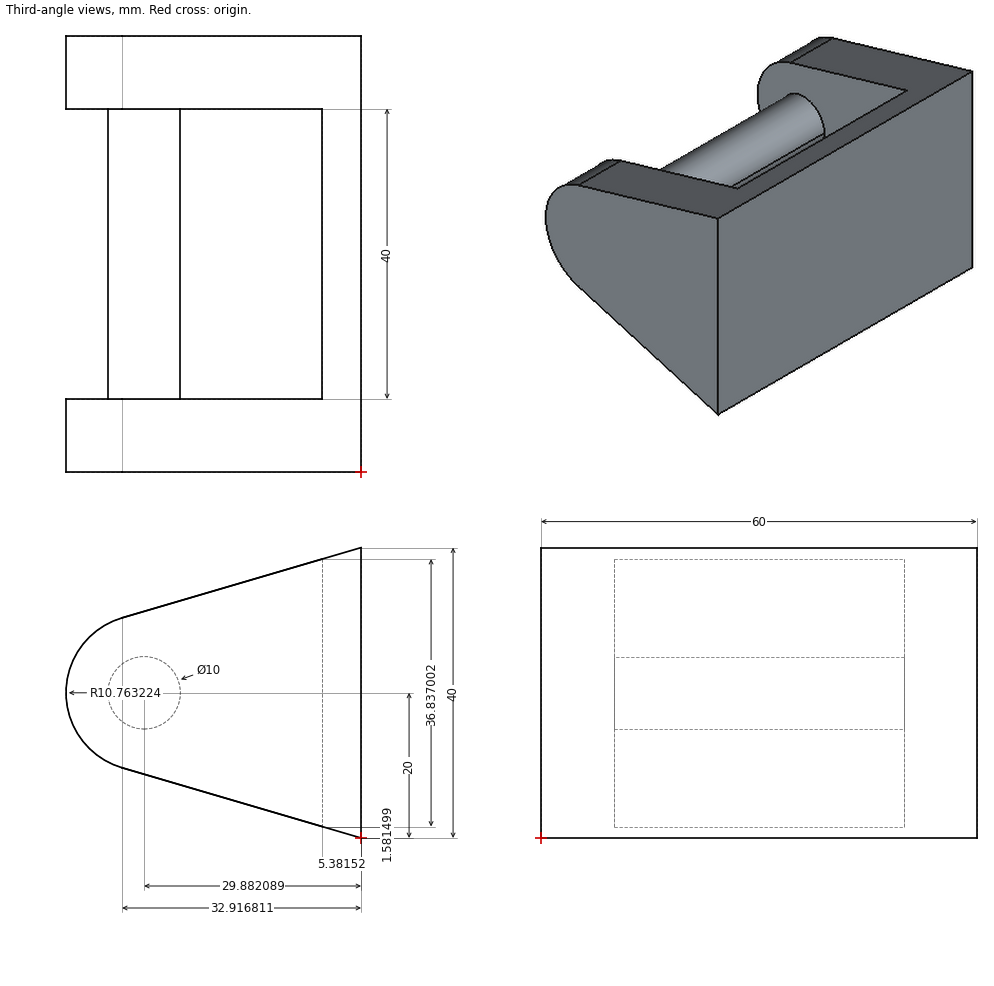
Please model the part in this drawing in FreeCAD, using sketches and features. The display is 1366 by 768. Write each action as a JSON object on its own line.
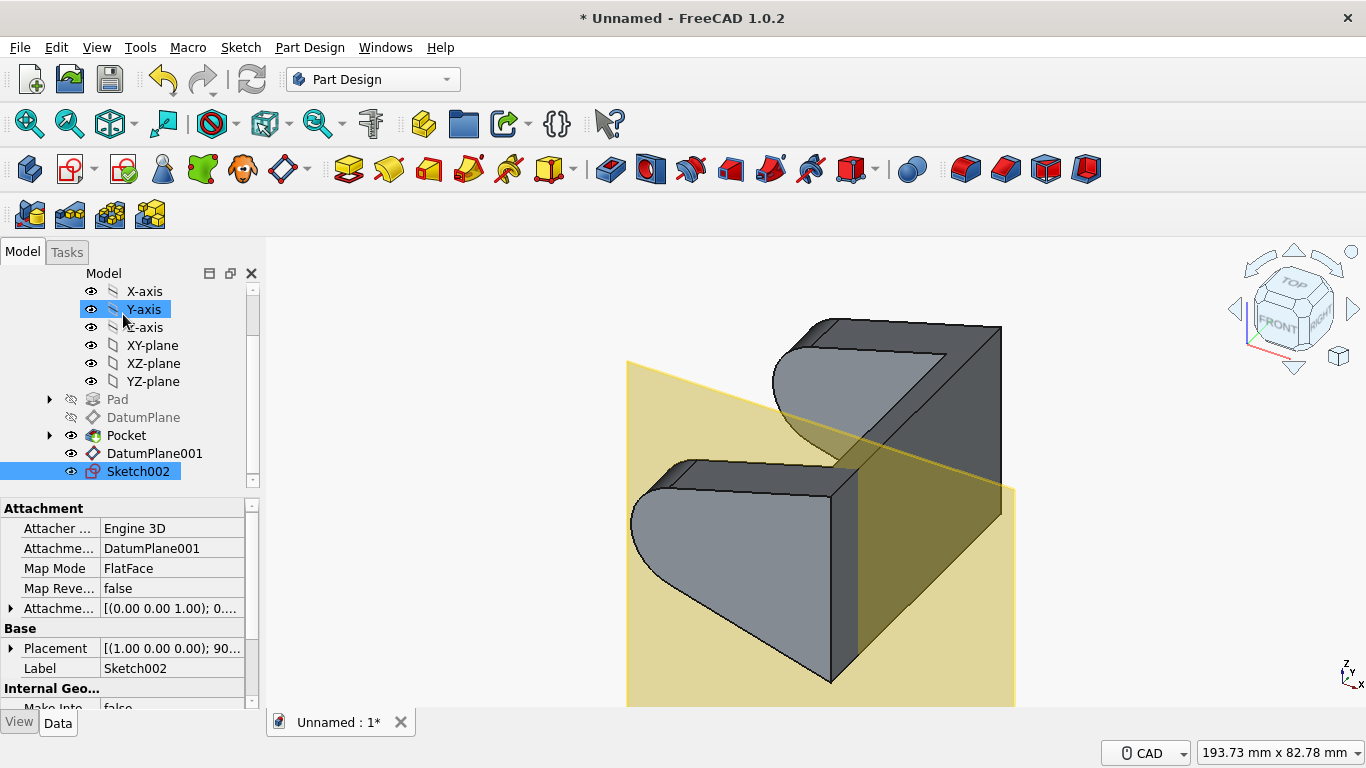
{"action": "left_click", "coordinate": [350, 170]}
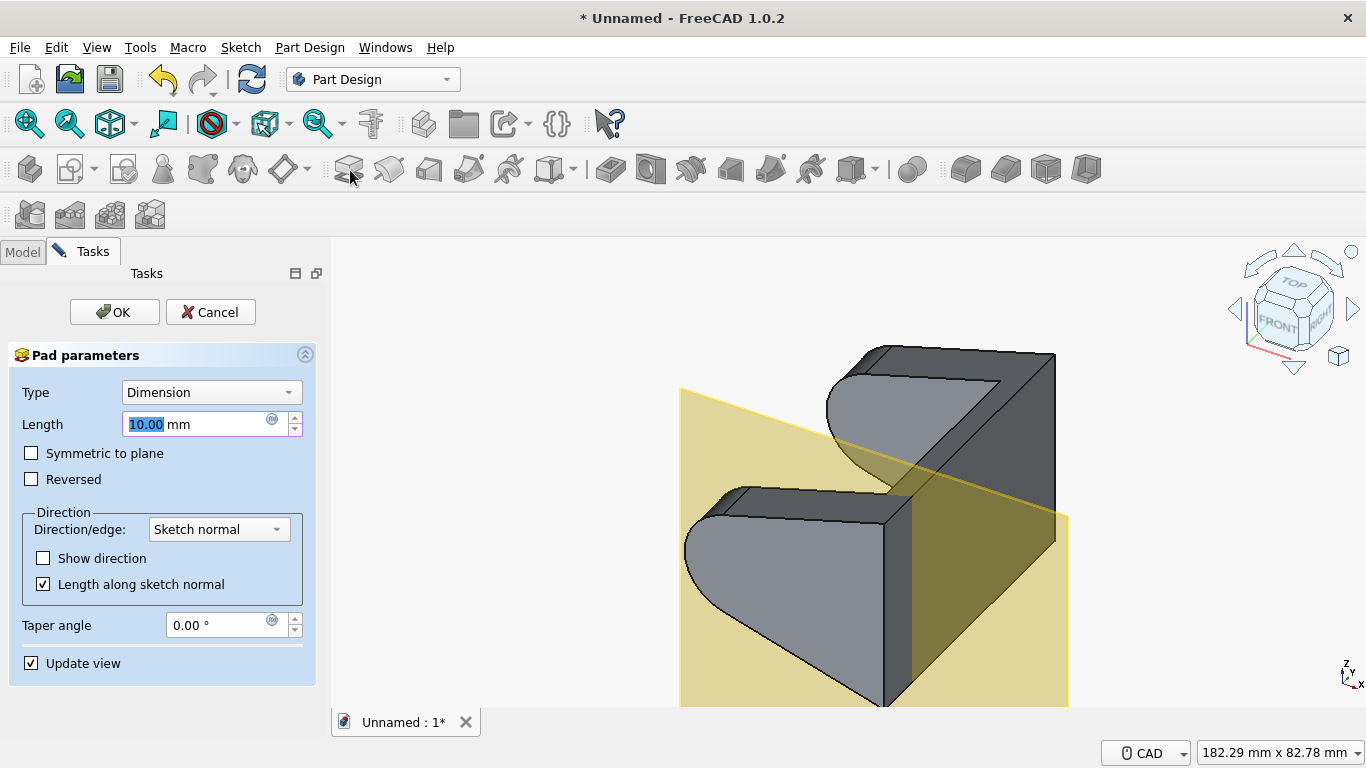
{"action": "left_click", "coordinate": [212, 392]}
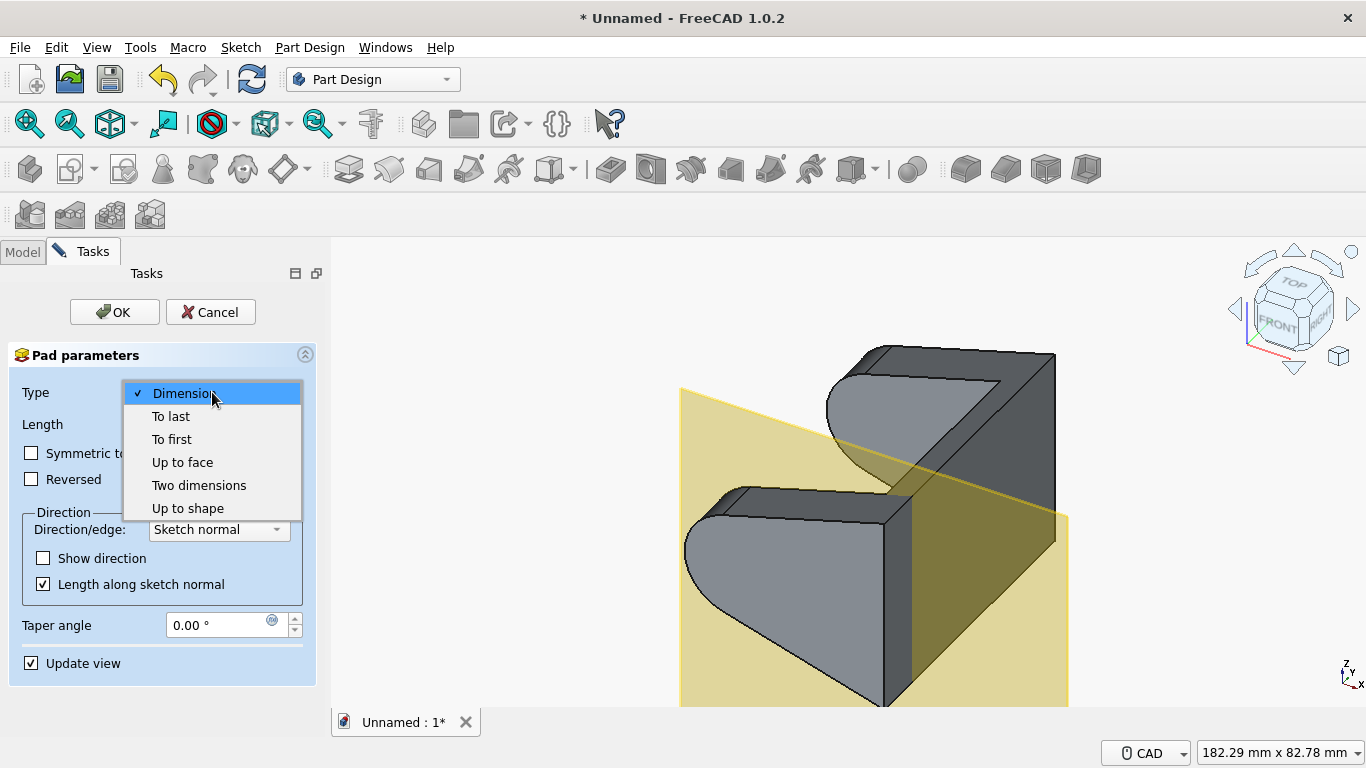
{"action": "left_click", "coordinate": [212, 440]}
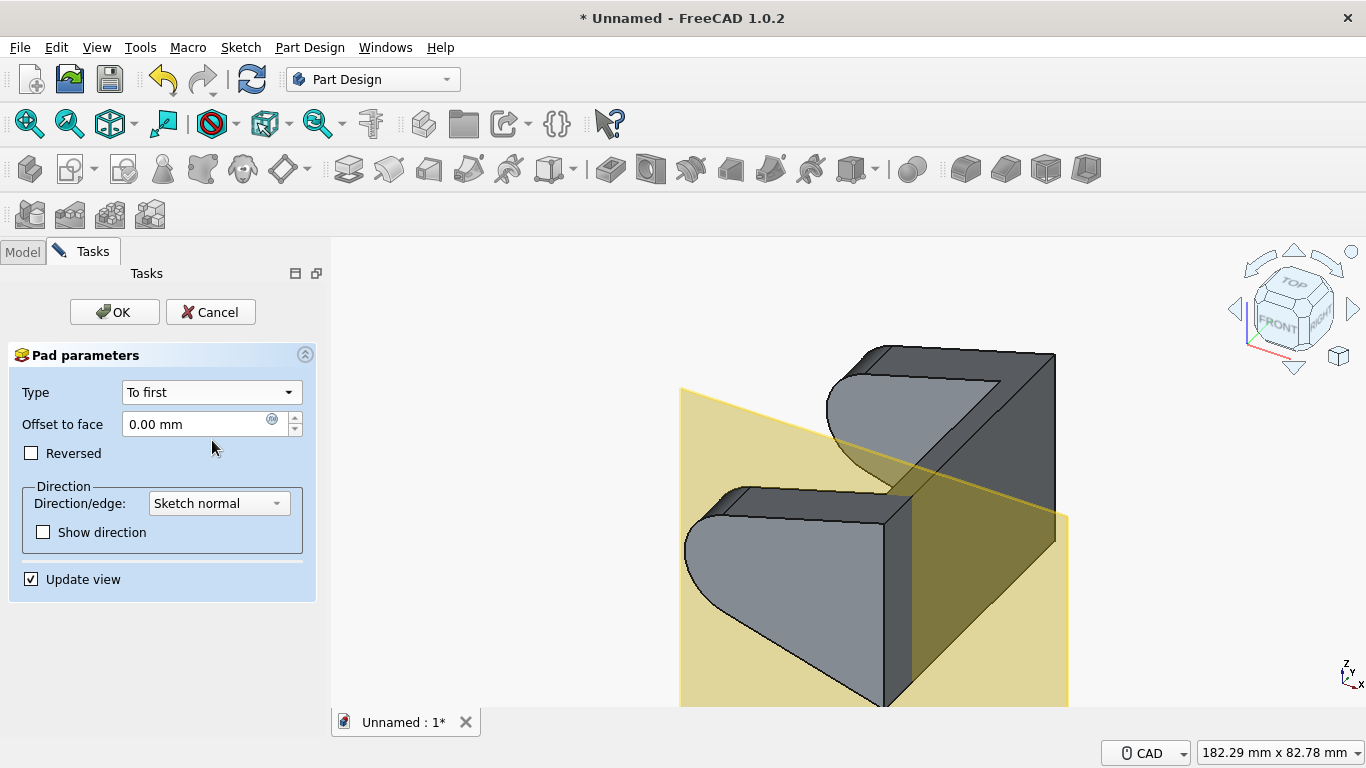
{"action": "left_click", "coordinate": [30, 453]}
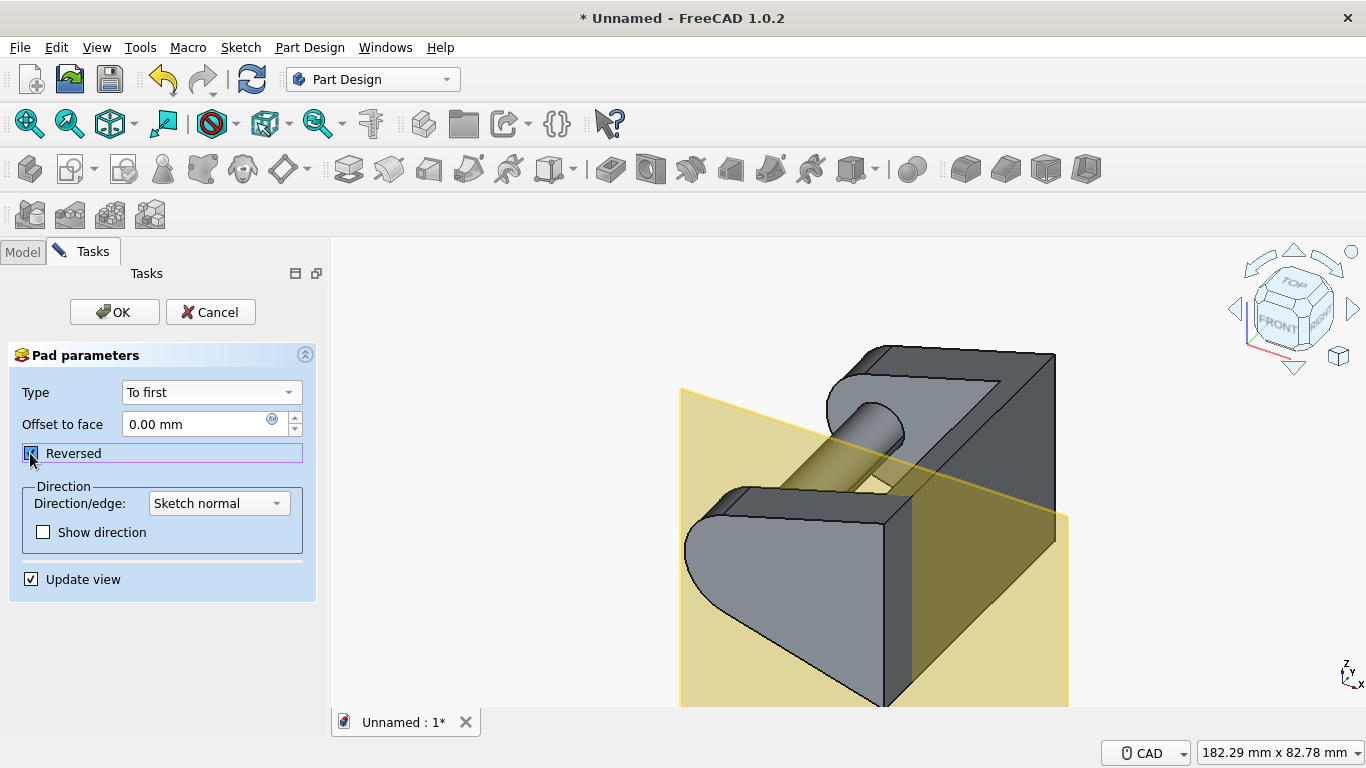
{"action": "left_click", "coordinate": [115, 312]}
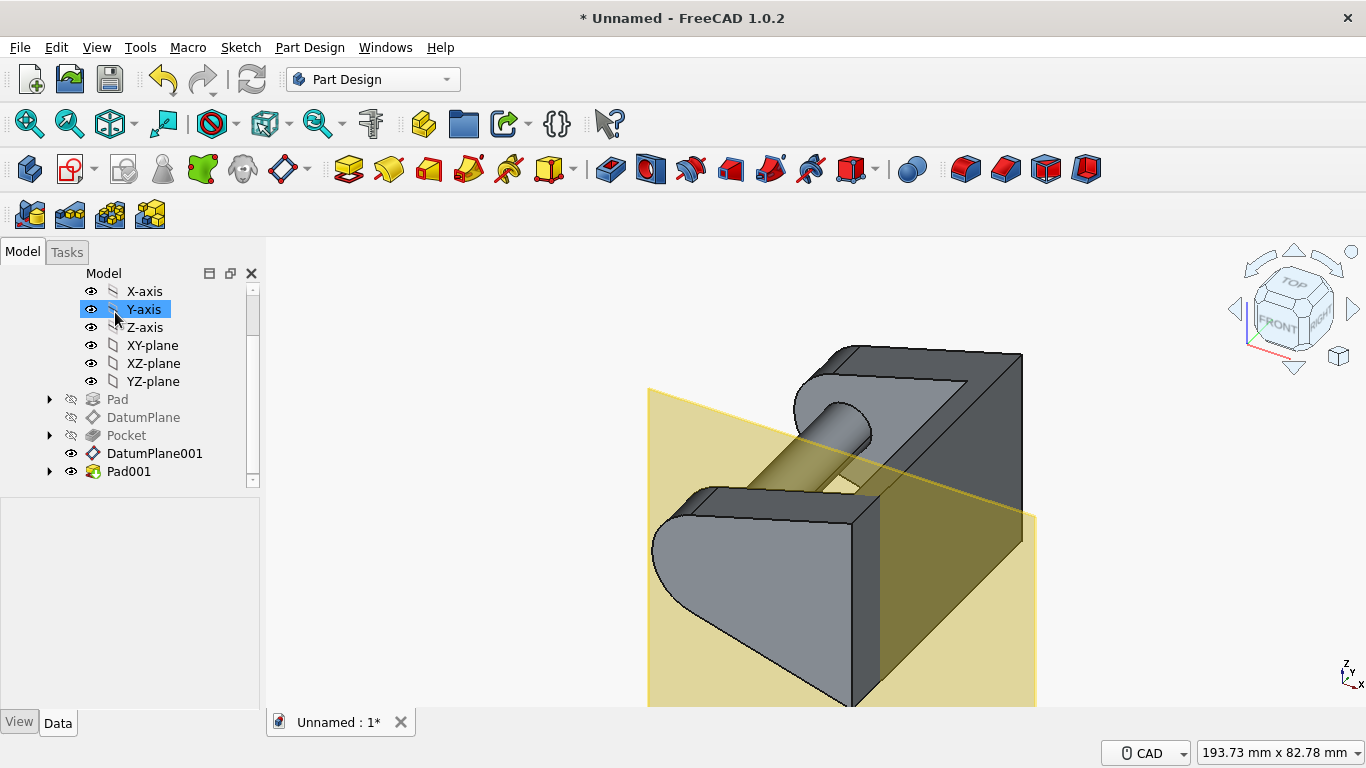
{"action": "left_click", "coordinate": [116, 453]}
{"action": "key", "text": "space"}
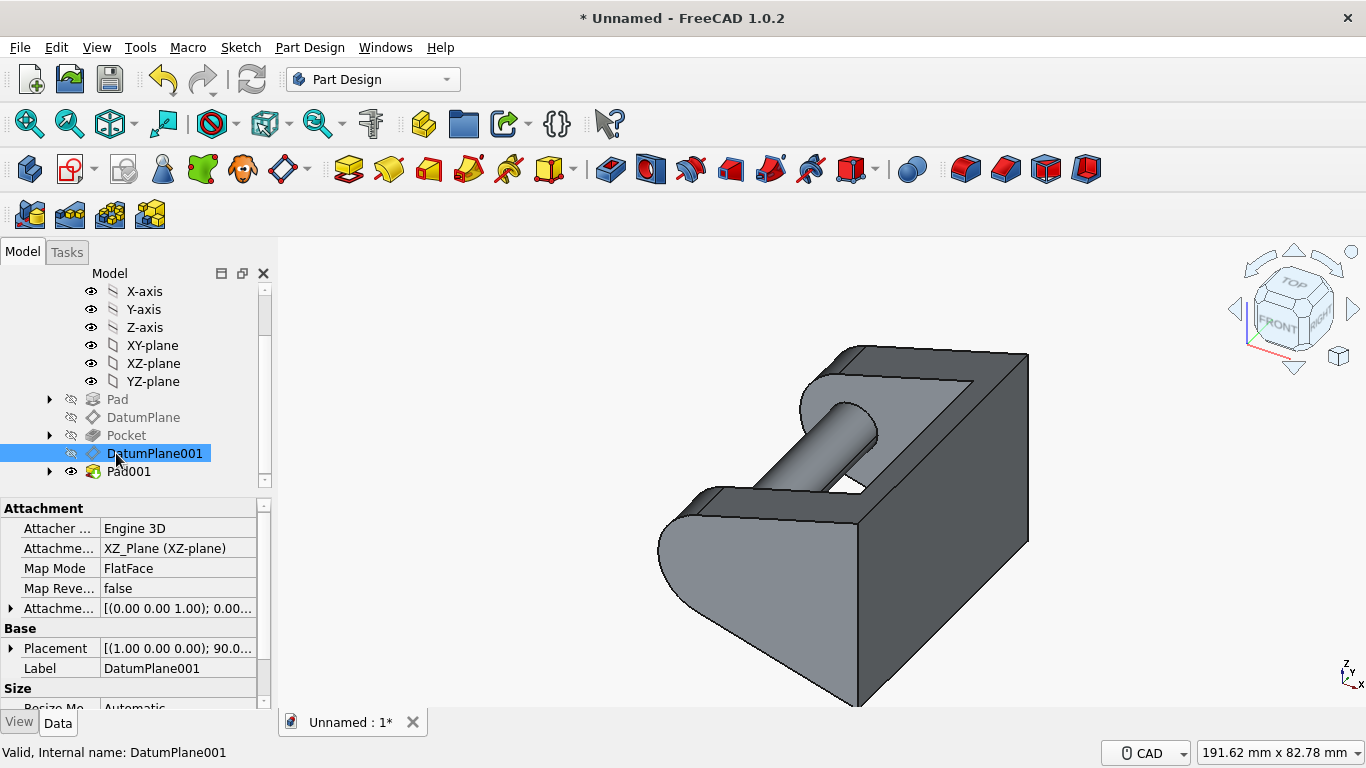
{"action": "key", "text": "0"}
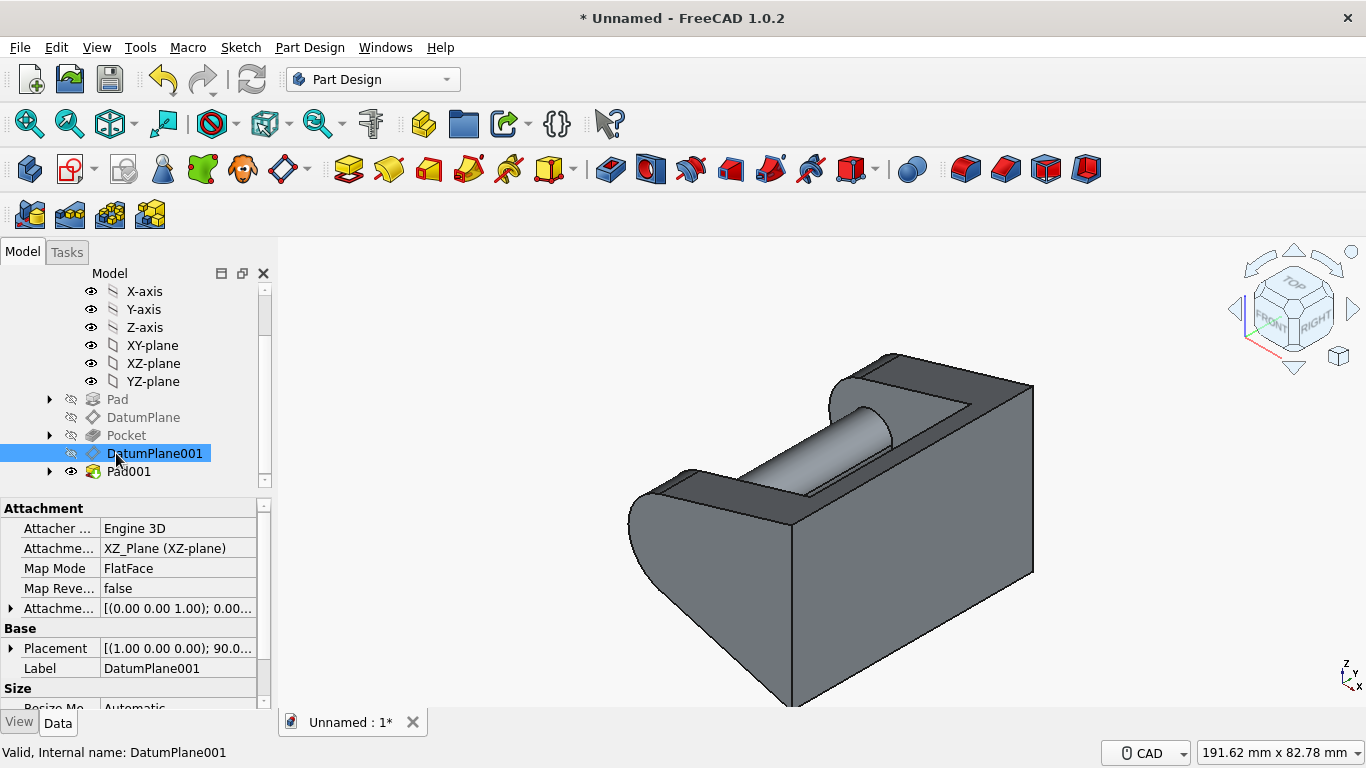
{"action": "left_click", "coordinate": [30, 124]}